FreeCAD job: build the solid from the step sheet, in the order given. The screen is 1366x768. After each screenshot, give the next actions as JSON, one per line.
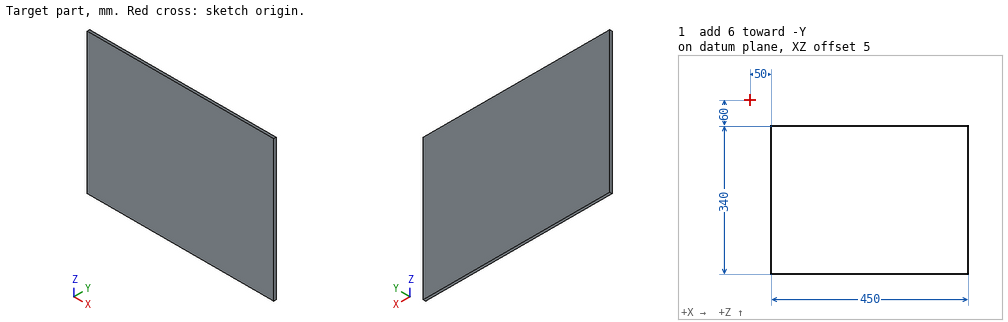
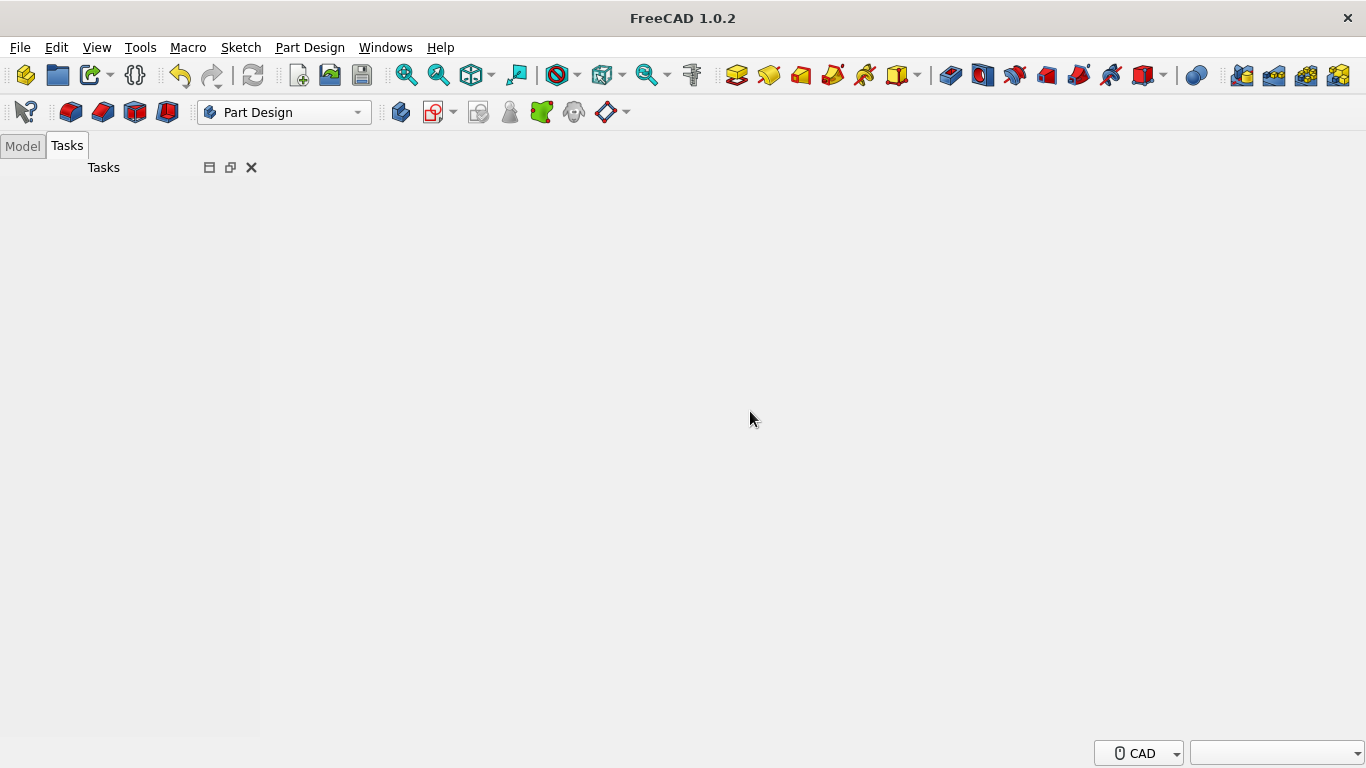
{"action": "key", "text": "ctrl+n"}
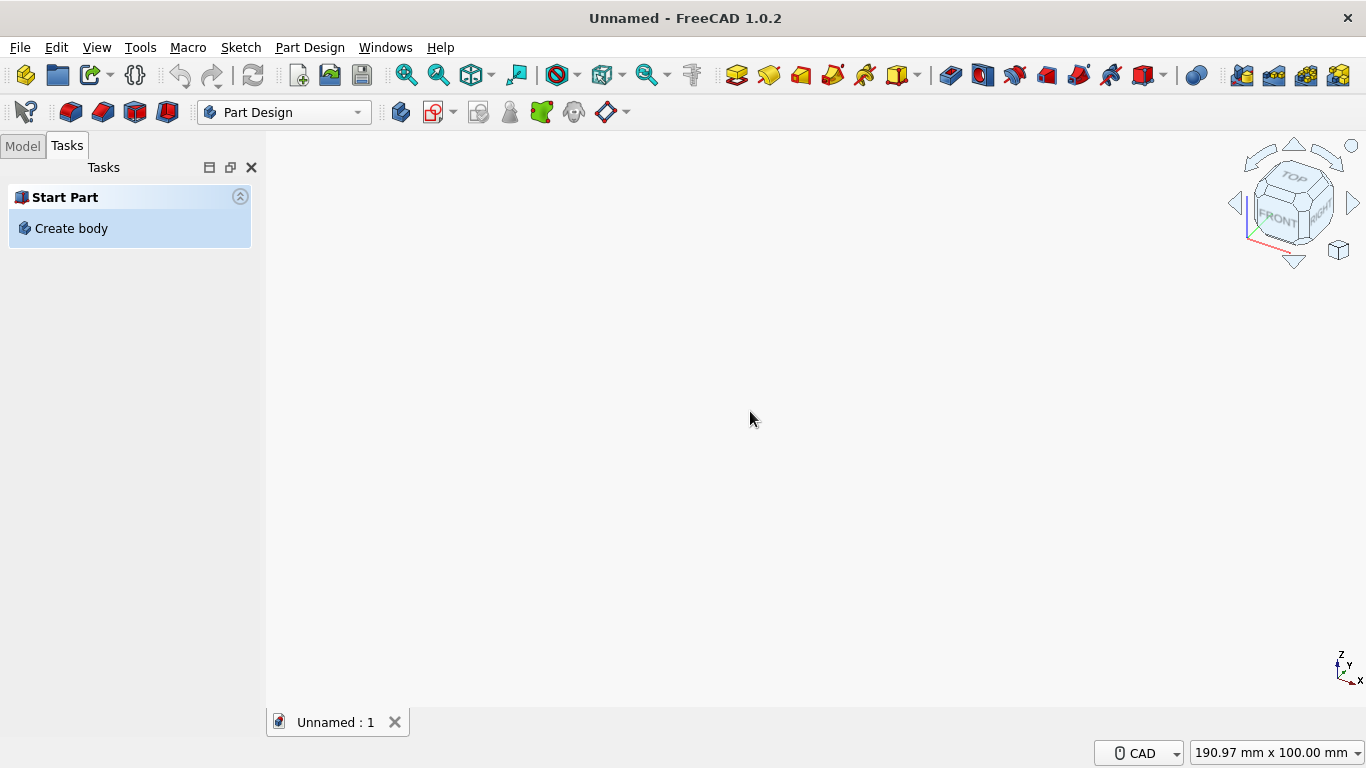
{"action": "left_click", "coordinate": [402, 112]}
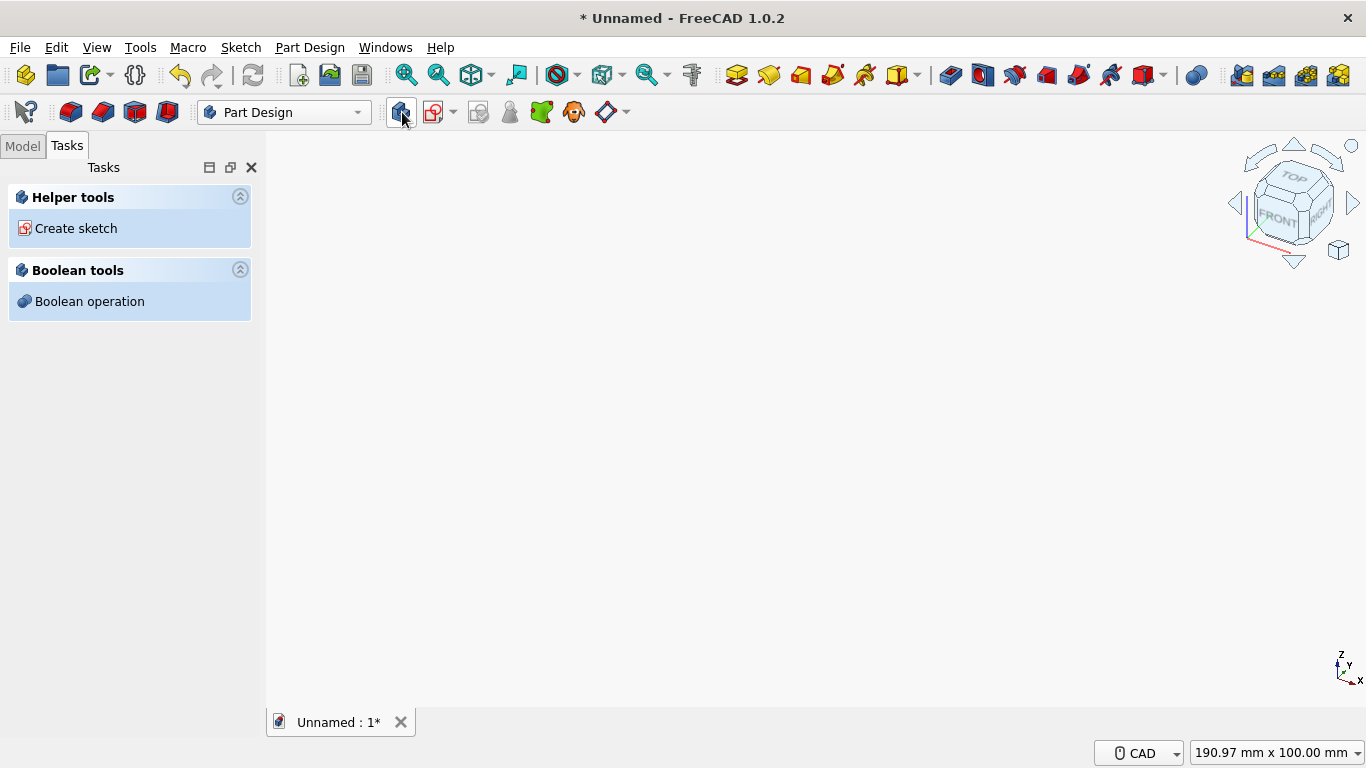
{"action": "left_click", "coordinate": [23, 145]}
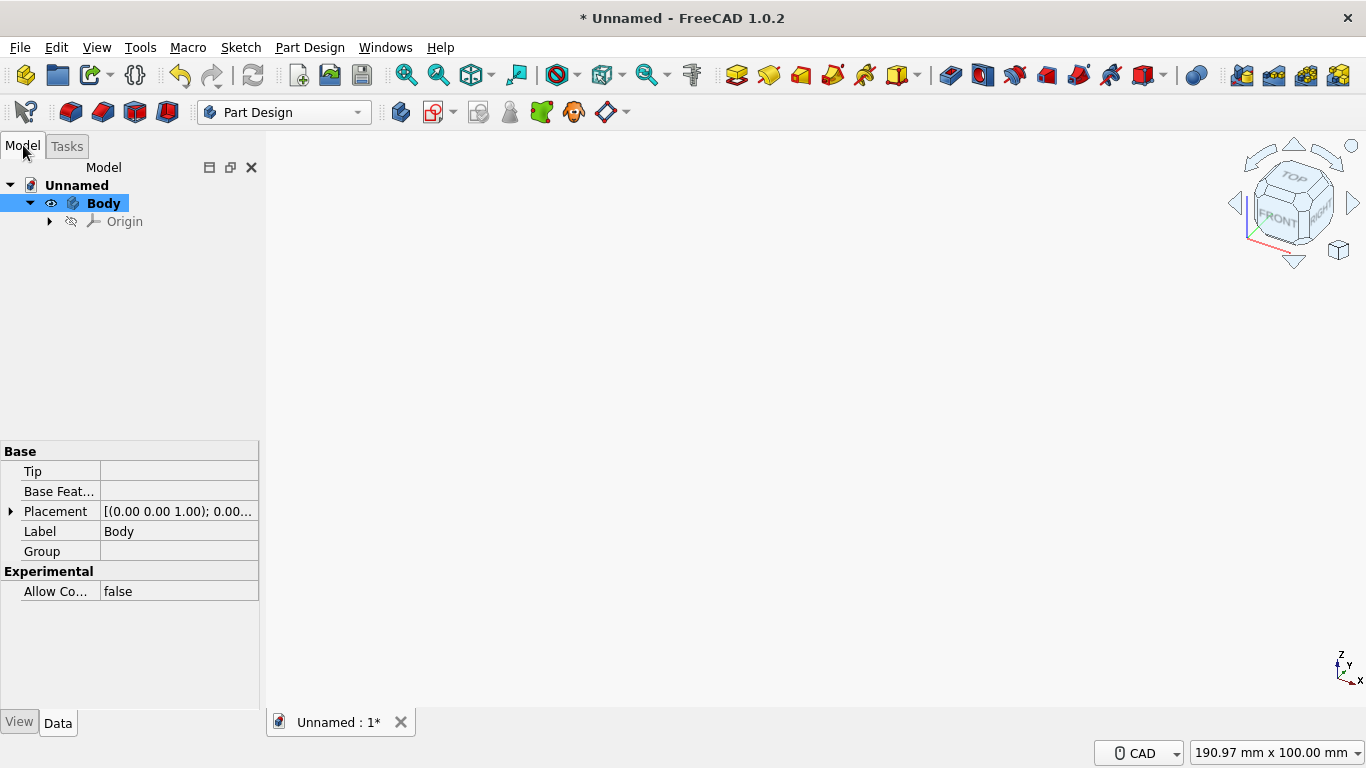
{"action": "left_click", "coordinate": [50, 221]}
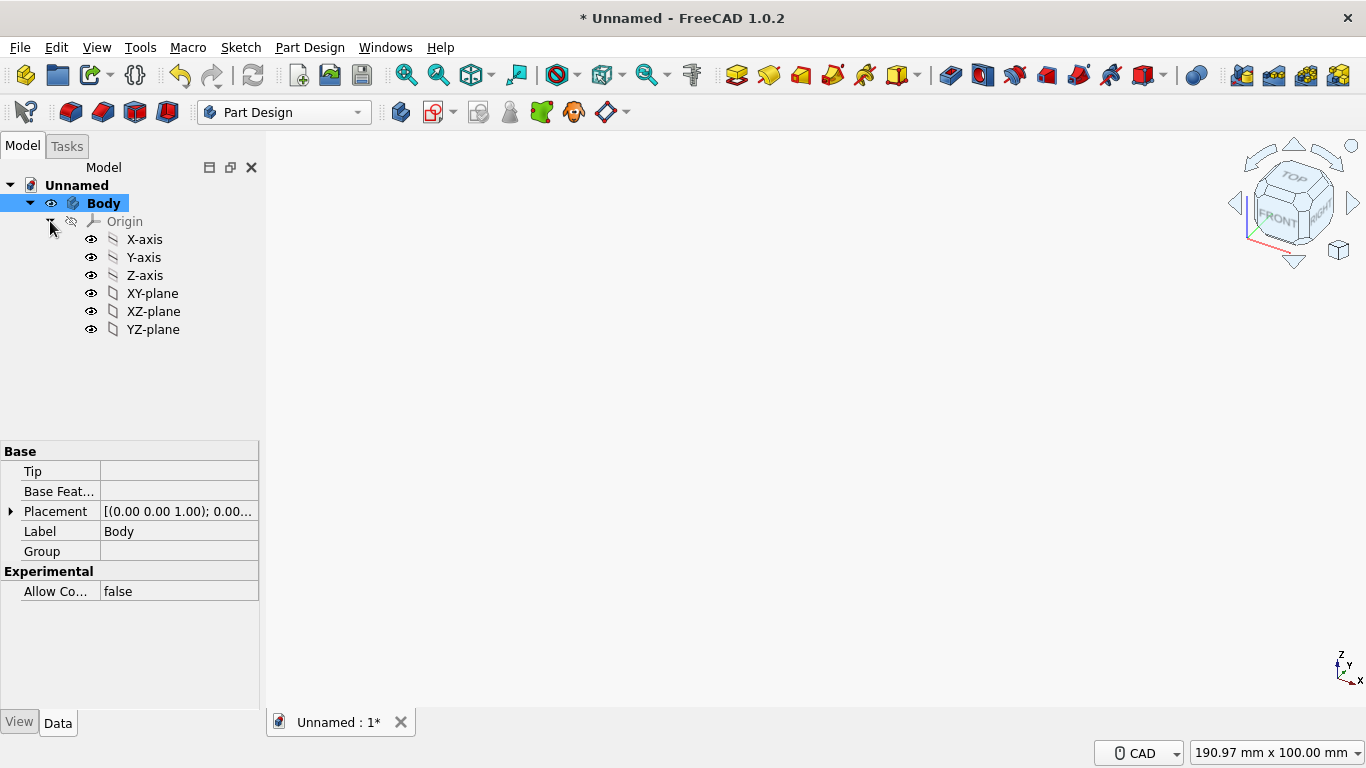
{"action": "left_click", "coordinate": [136, 311]}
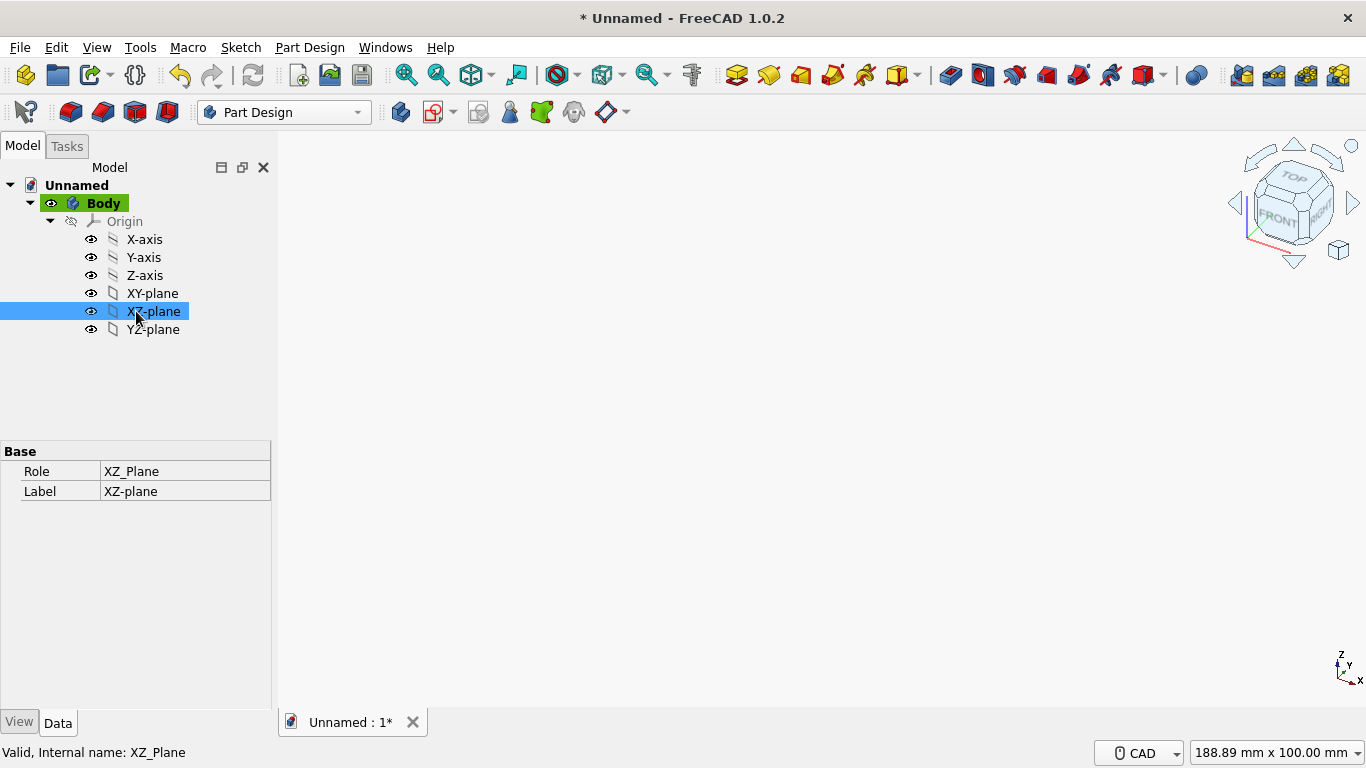
{"action": "left_click", "coordinate": [606, 112]}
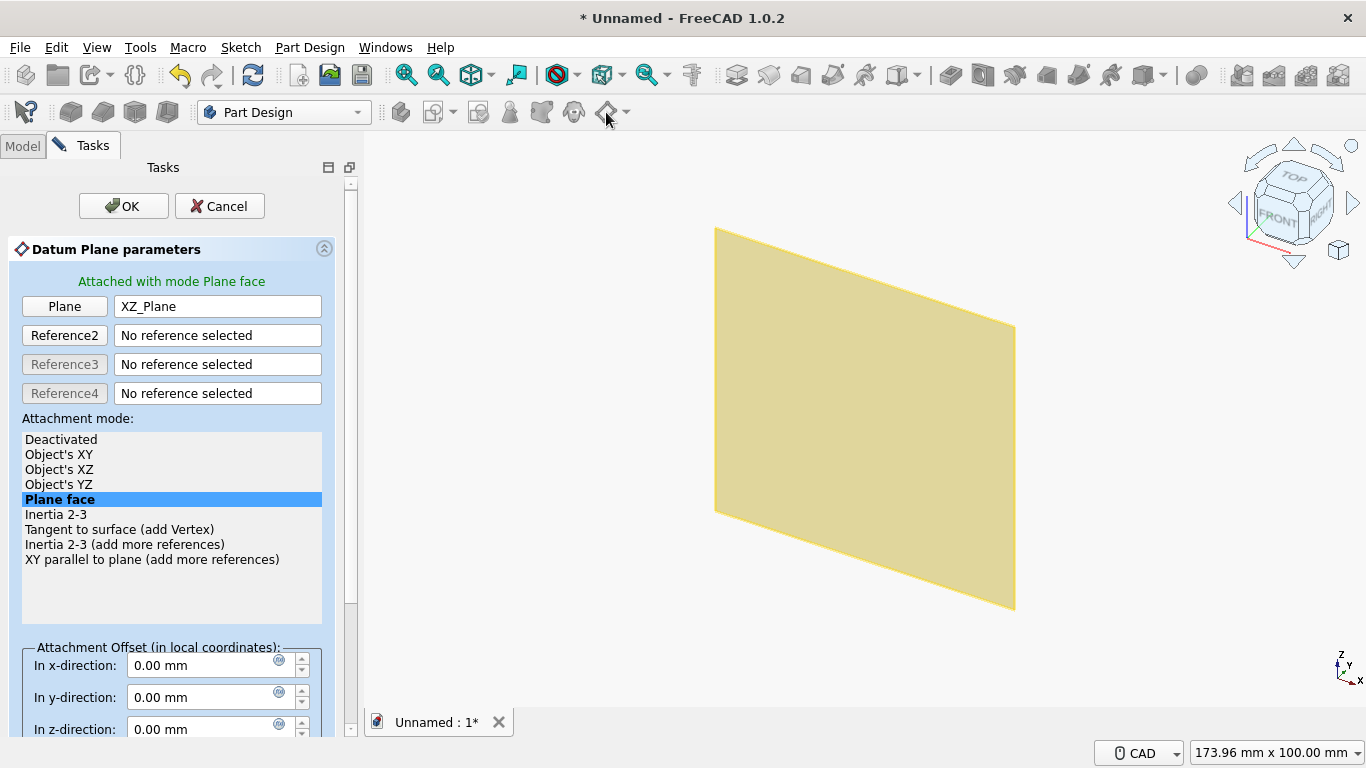
{"action": "scroll", "coordinate": [351, 456], "scroll_direction": "down", "scroll_amount": 2}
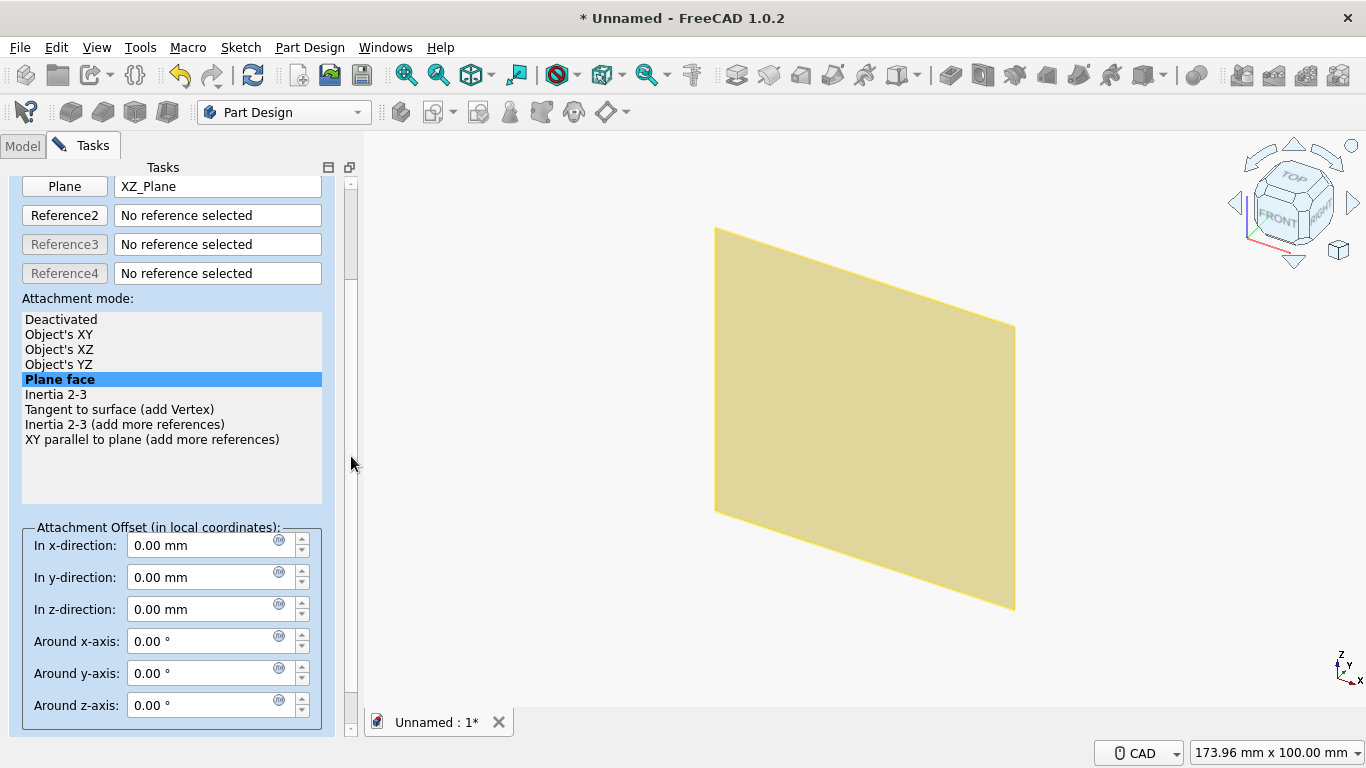
{"action": "triple_click", "coordinate": [210, 609]}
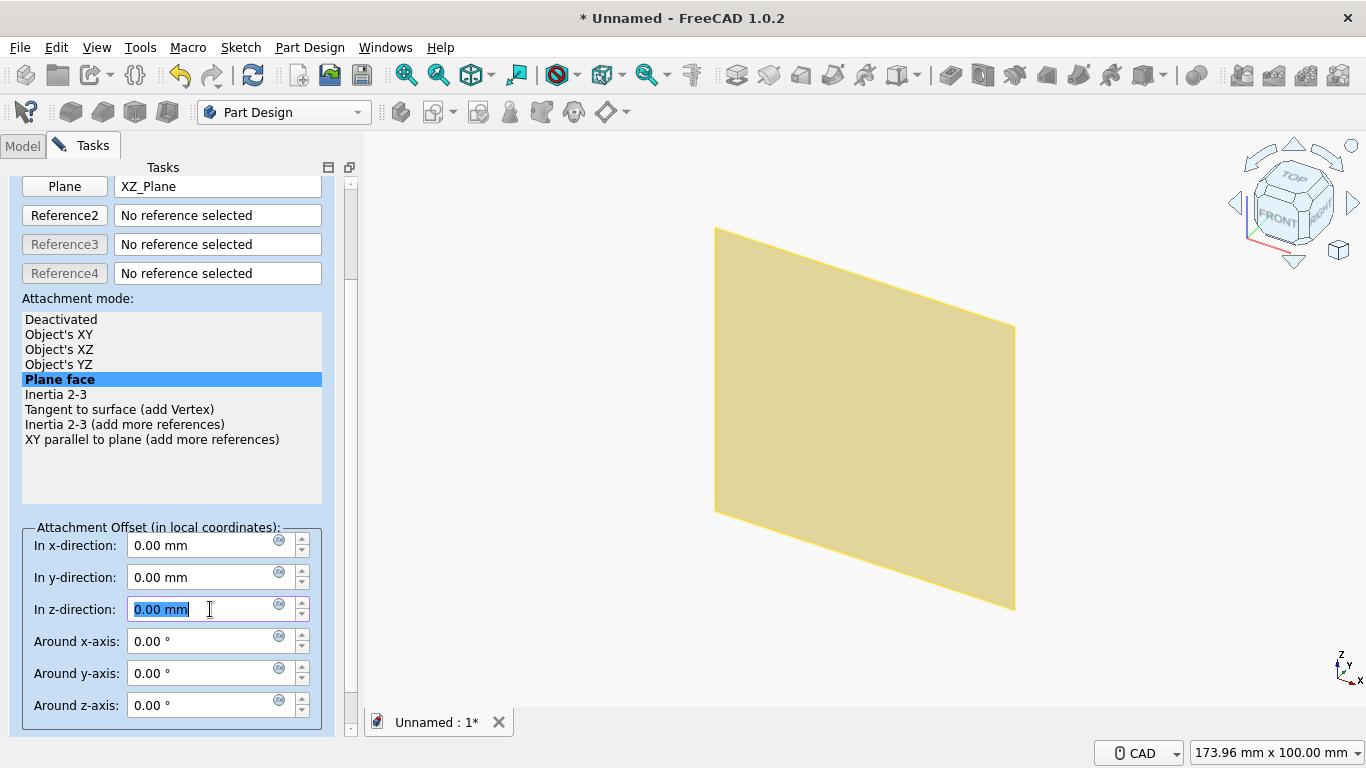
{"action": "type", "text": "5"}
{"action": "key", "text": "Tab"}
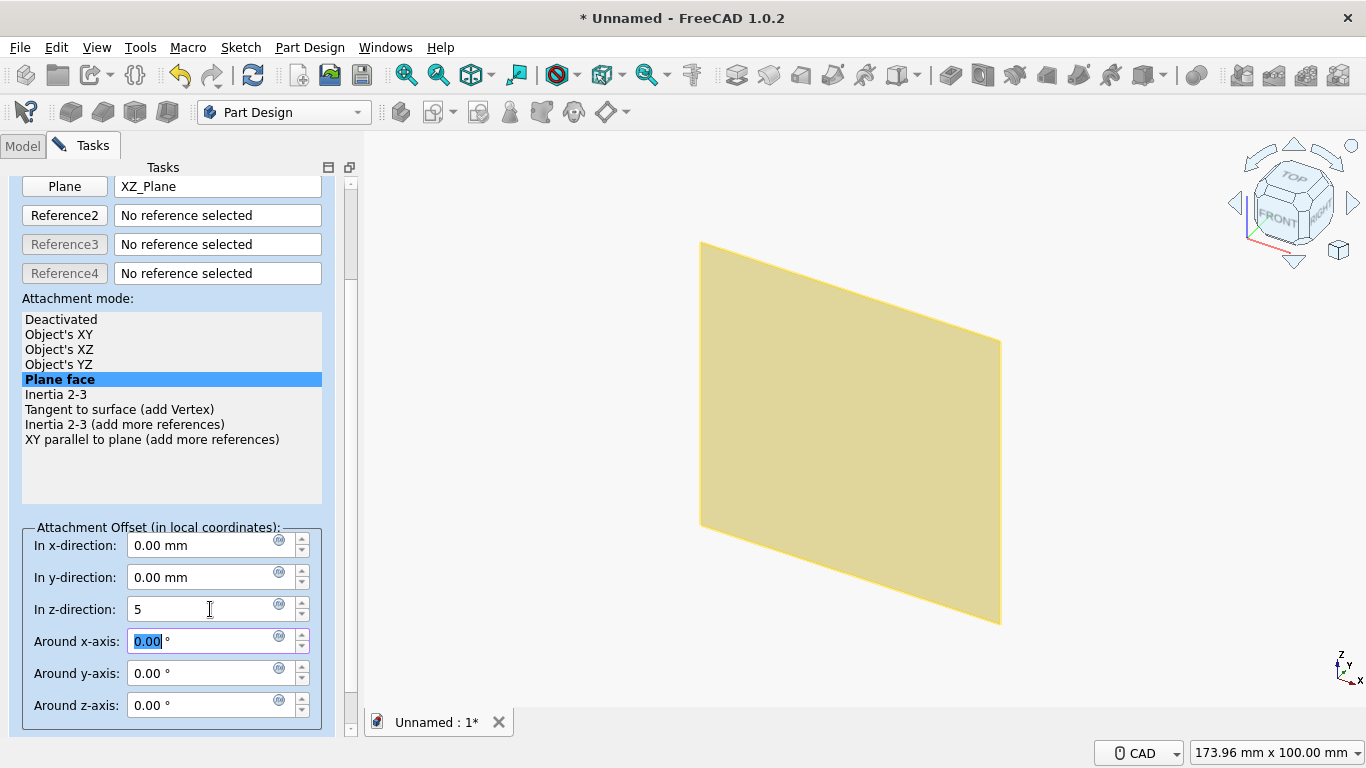
{"action": "scroll", "coordinate": [351, 456], "scroll_direction": "up", "scroll_amount": 3}